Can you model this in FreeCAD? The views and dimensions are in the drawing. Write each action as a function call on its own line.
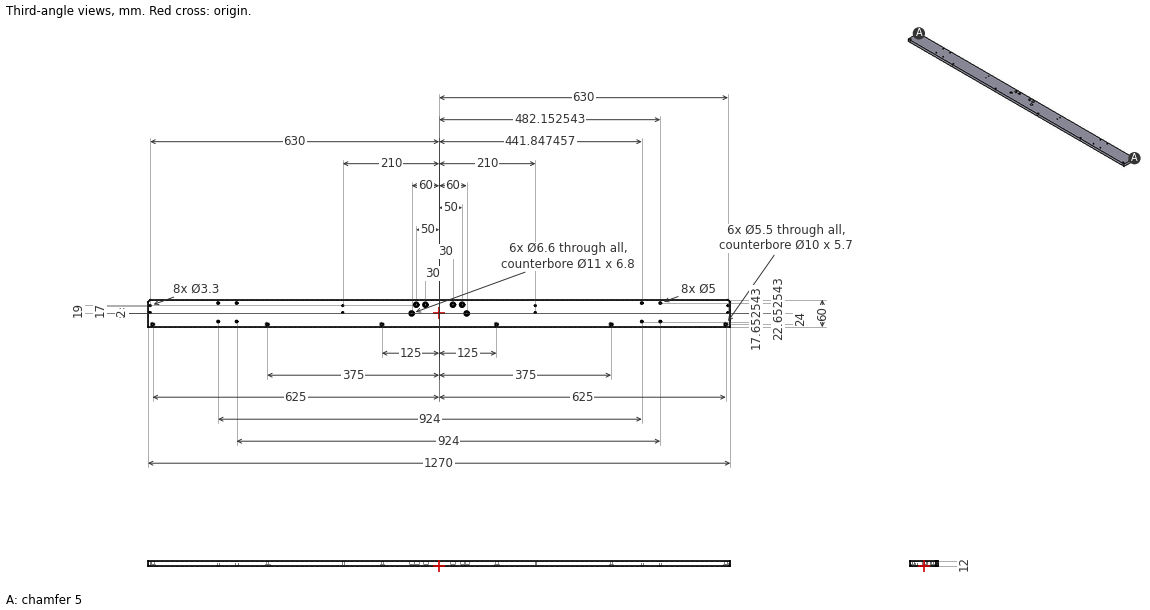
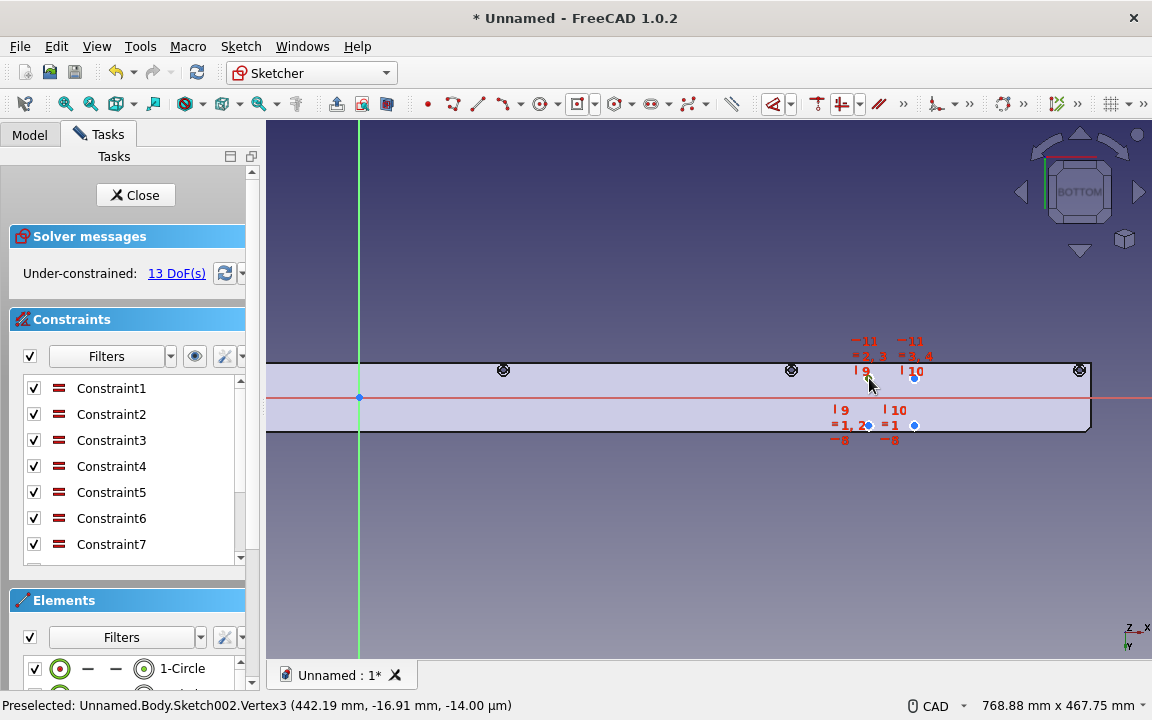
scroll(870, 380, down, 4)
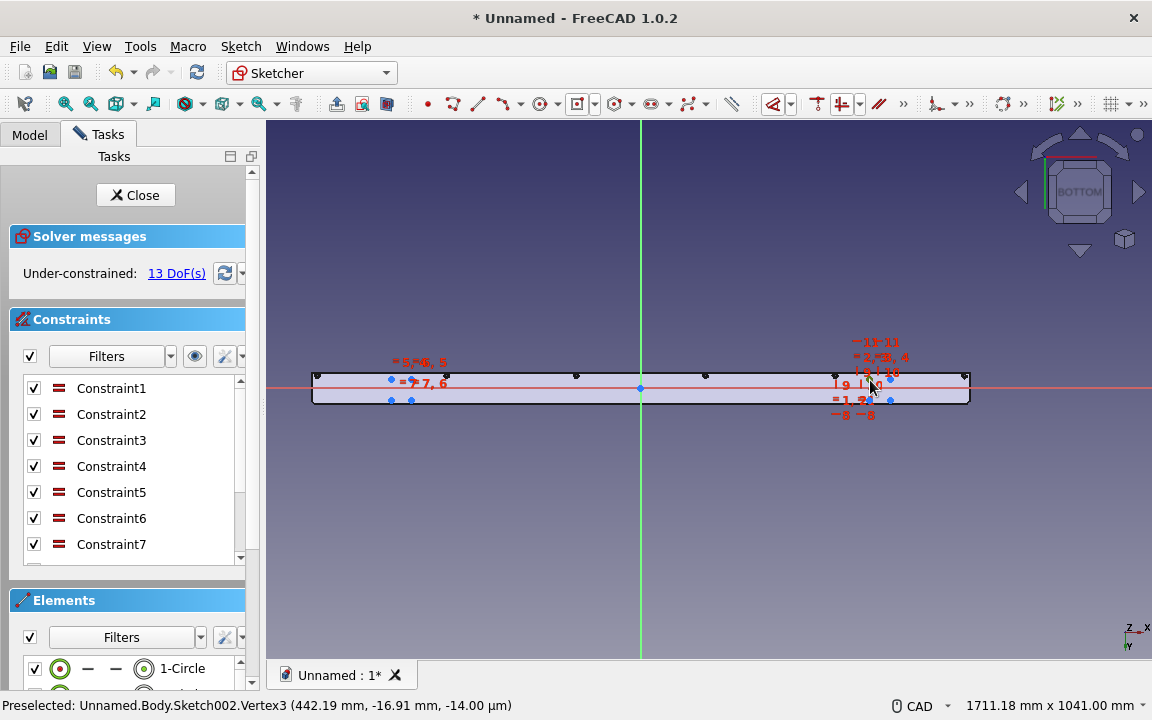
click(391, 380)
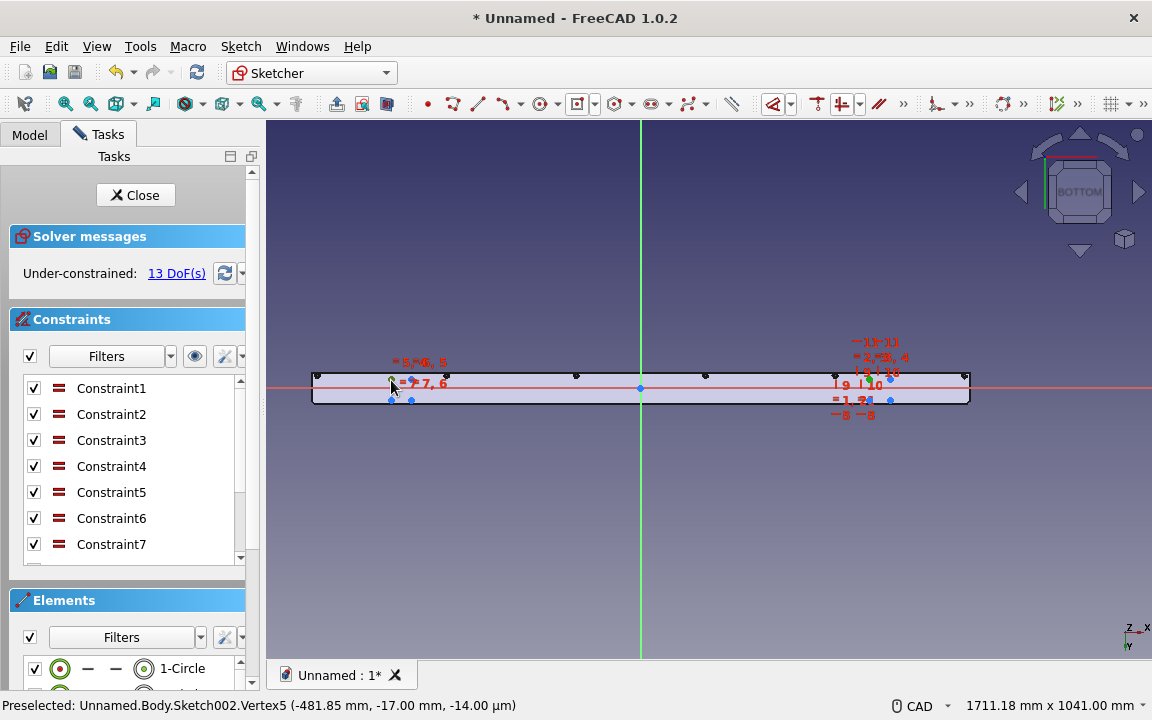
key(h)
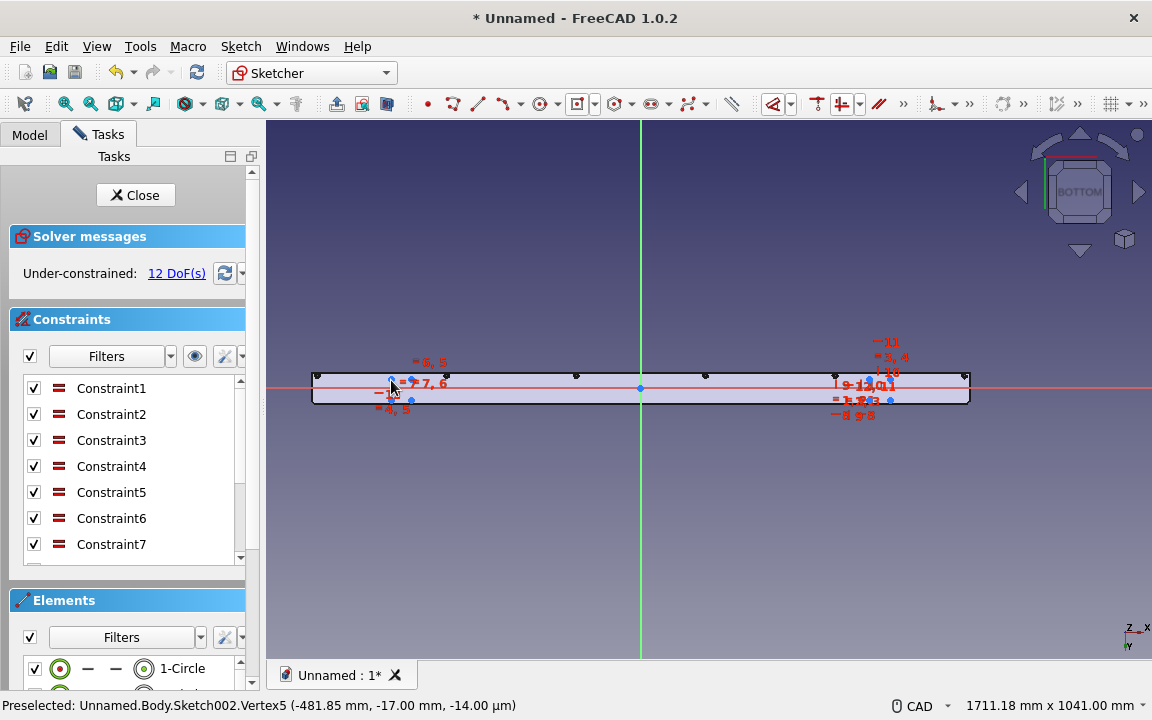
click(391, 380)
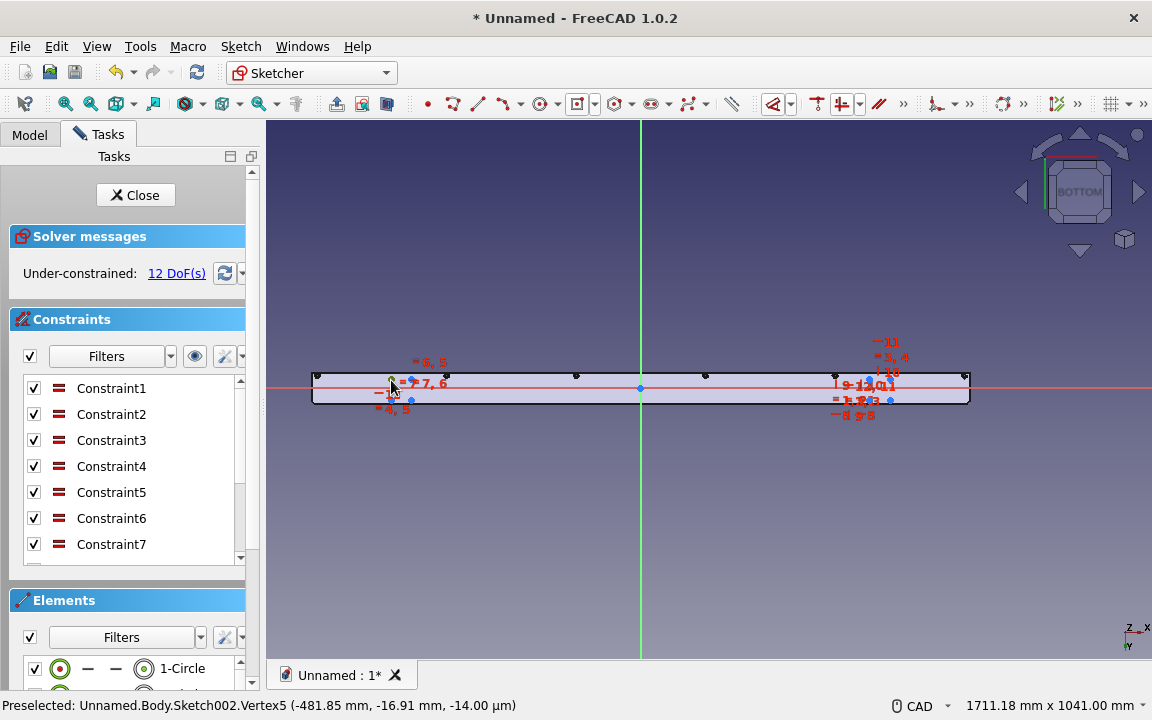
scroll(412, 380, up, 4)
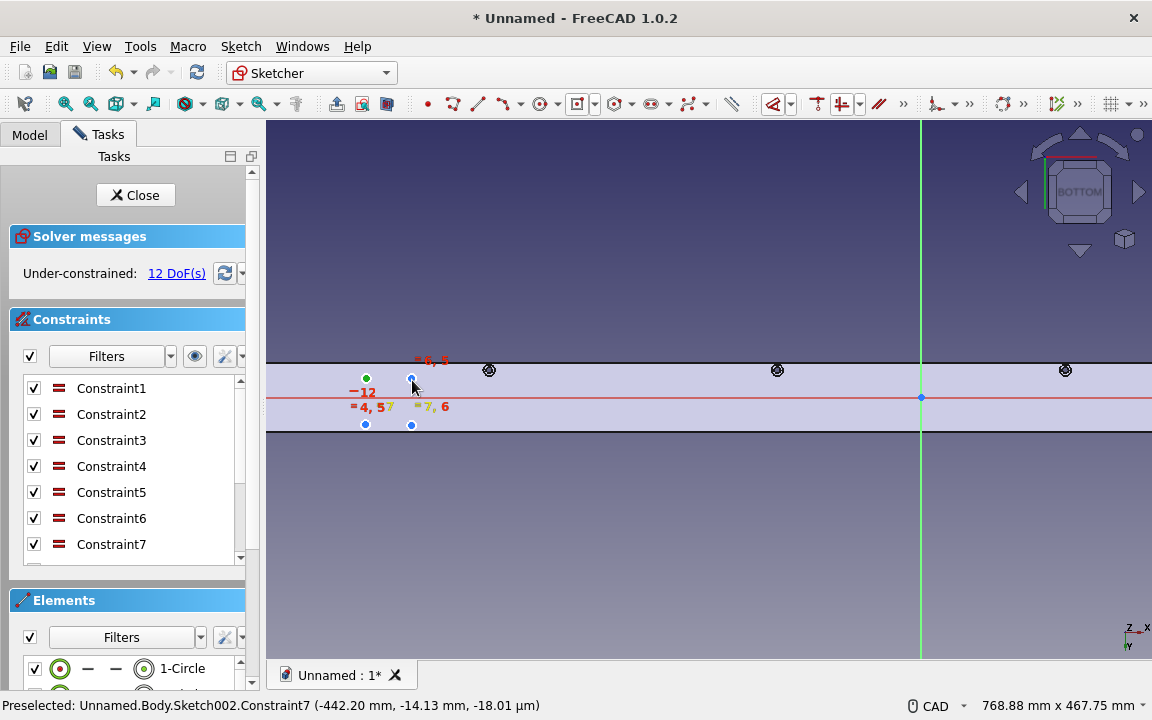
click(412, 379)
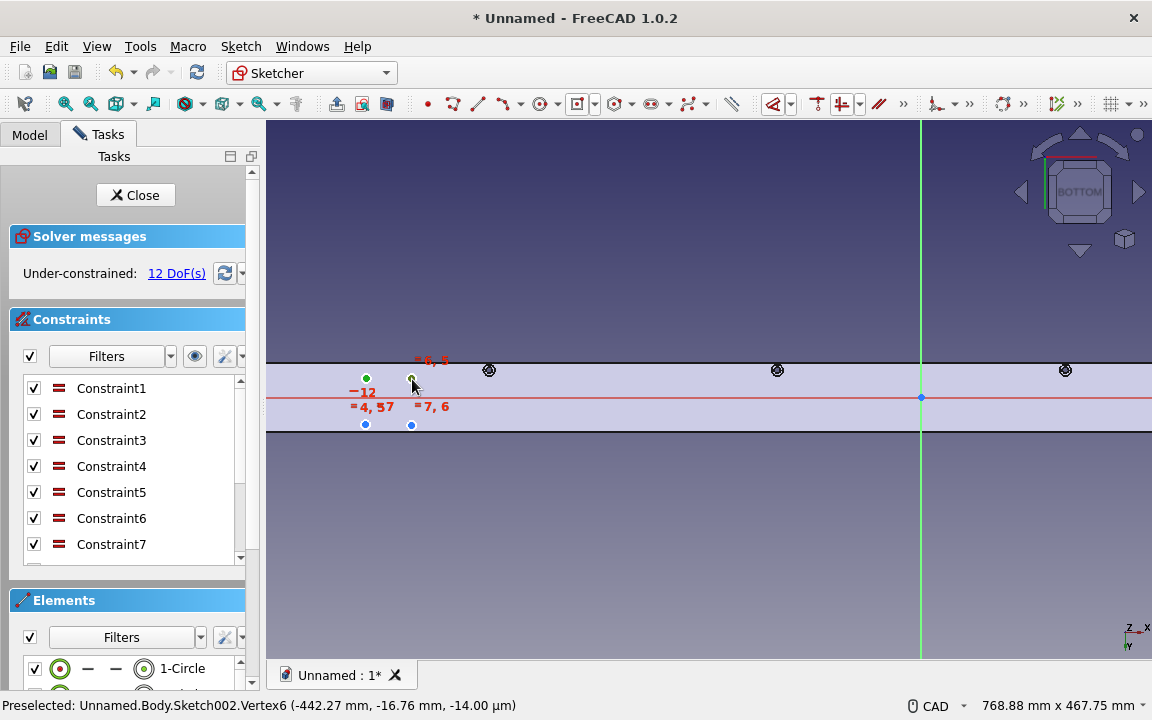
key(h)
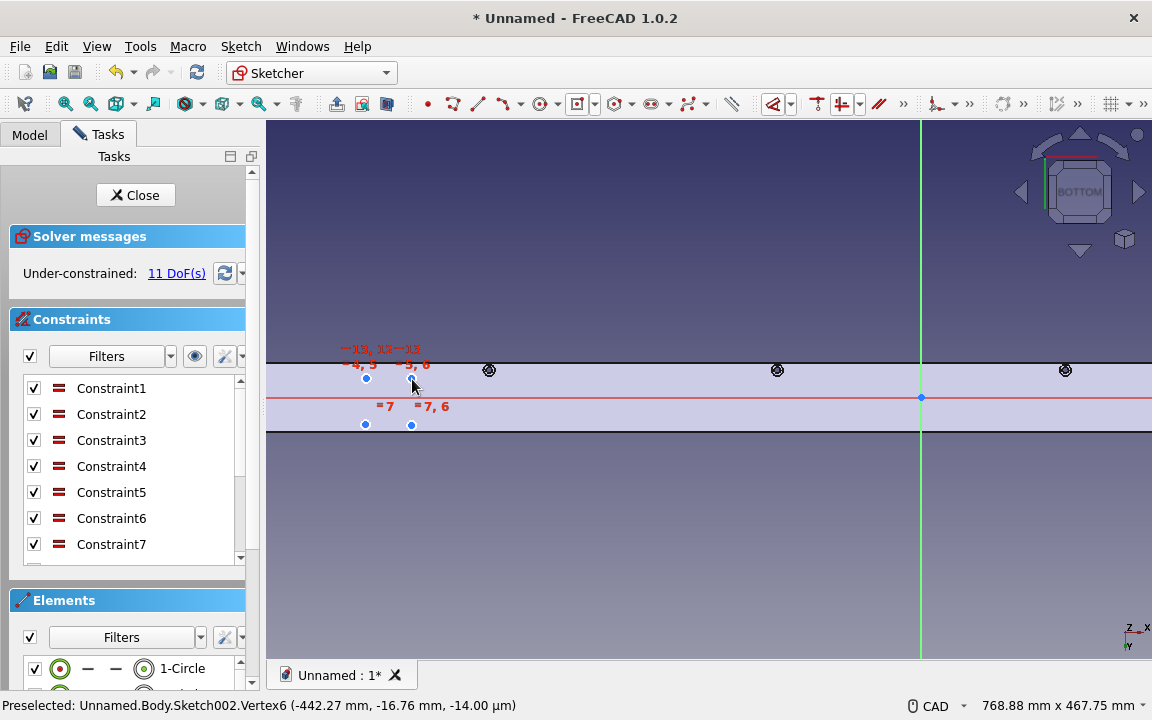
click(412, 378)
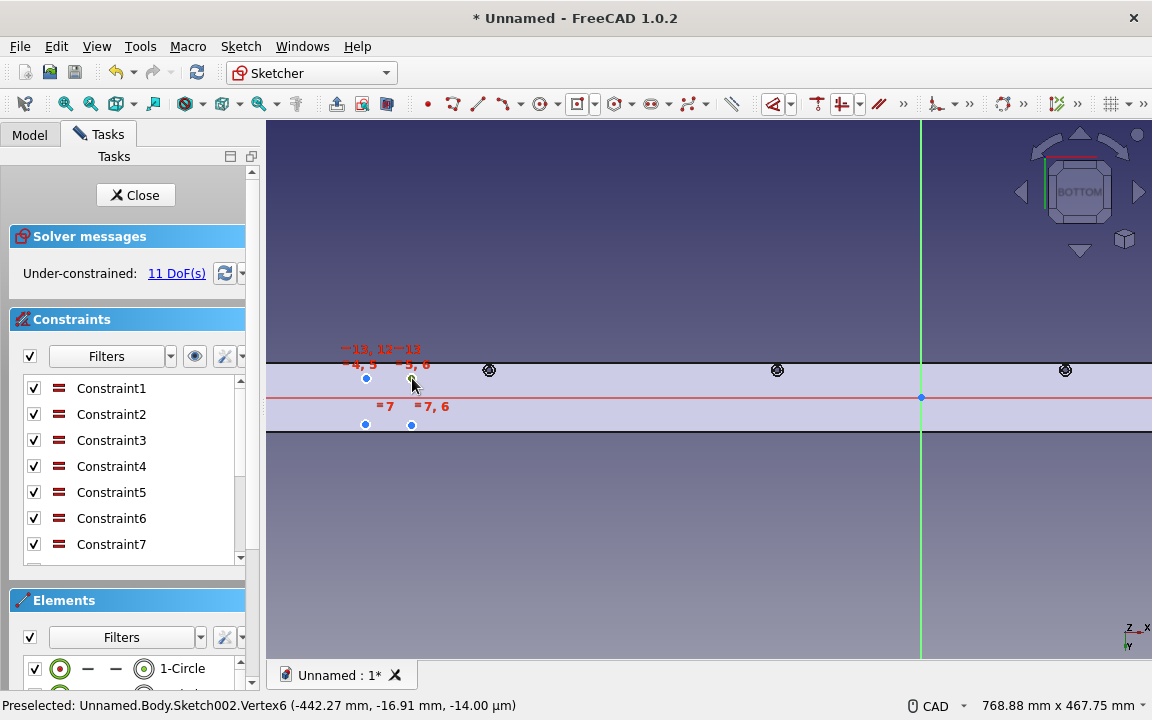
click(412, 425)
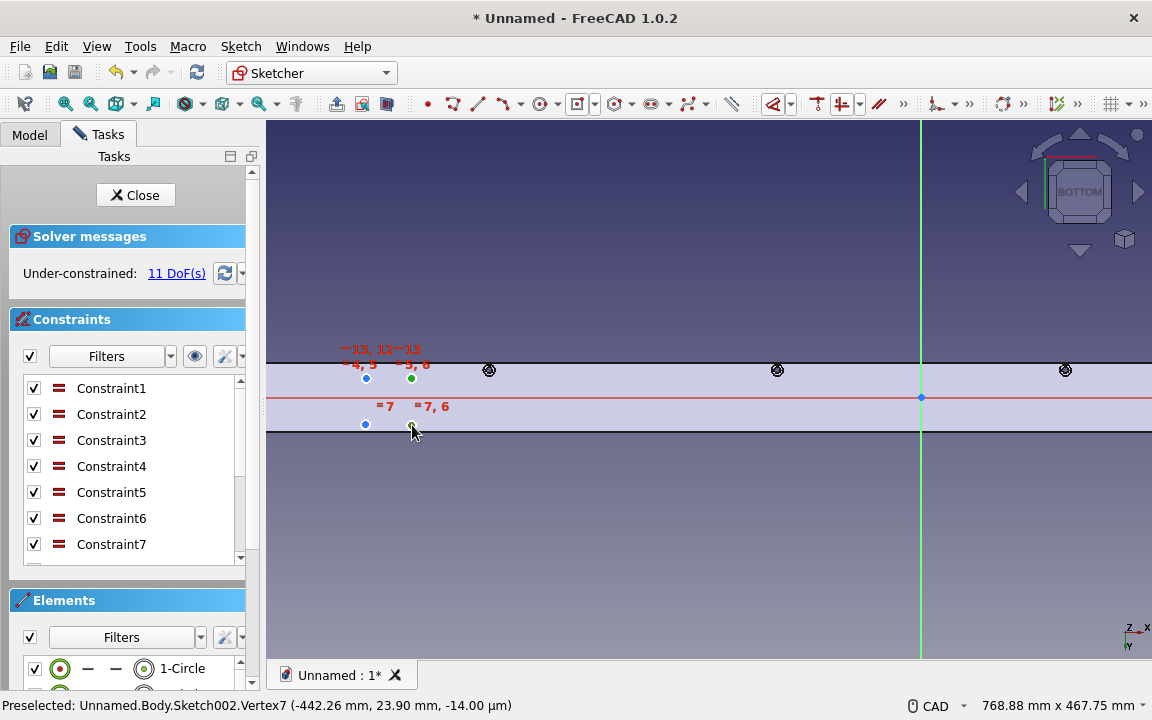
key(v)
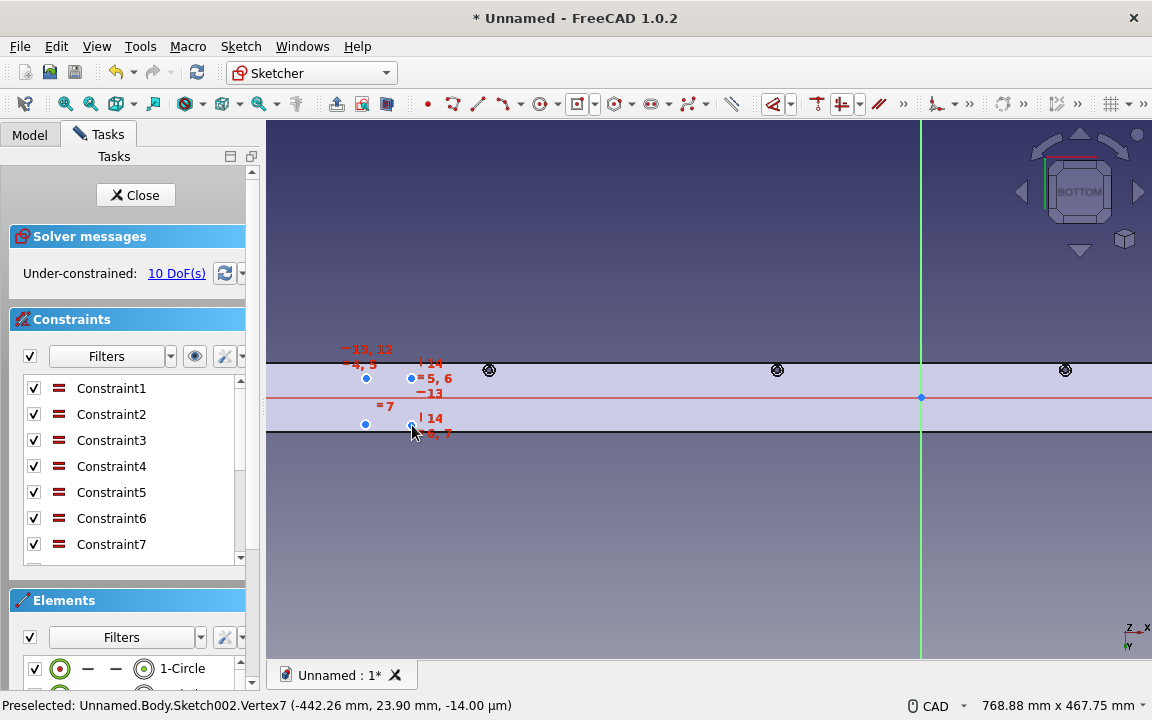
scroll(411, 380, down, 4)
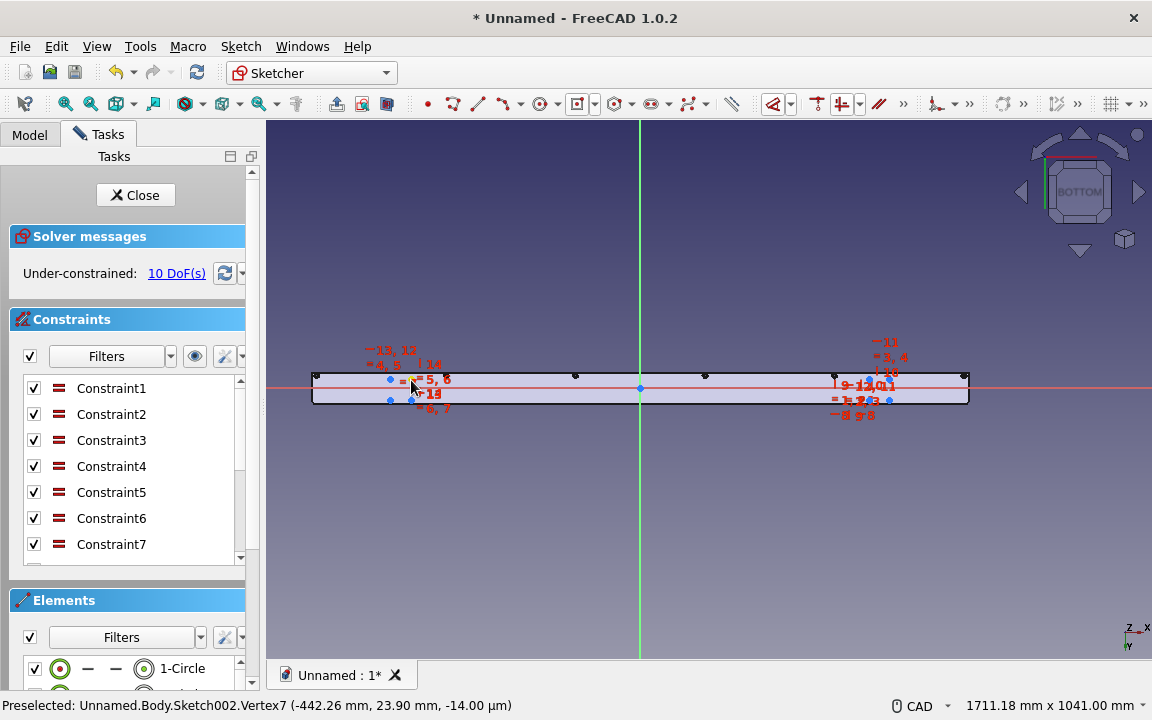
click(869, 401)